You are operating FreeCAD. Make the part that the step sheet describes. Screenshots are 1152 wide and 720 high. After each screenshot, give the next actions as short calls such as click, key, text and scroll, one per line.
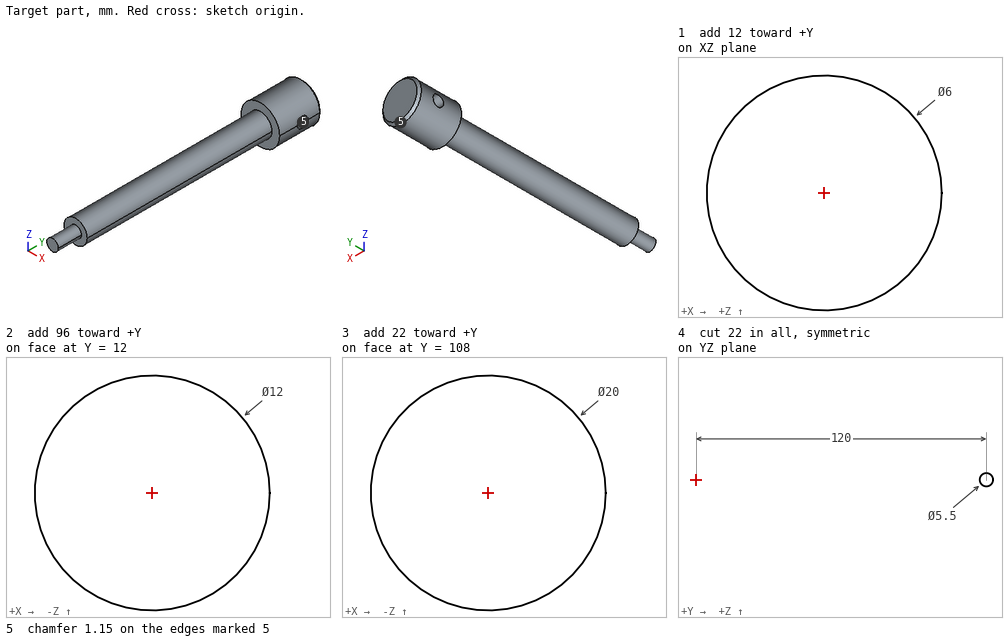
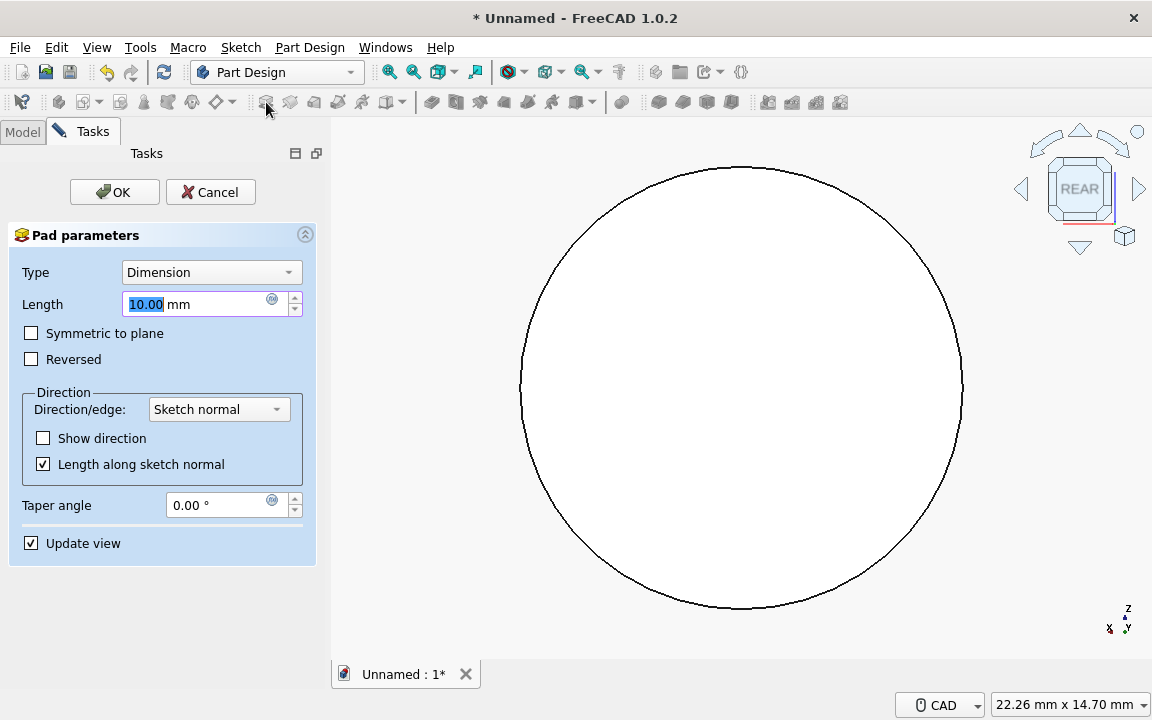
text(96)
key(Tab)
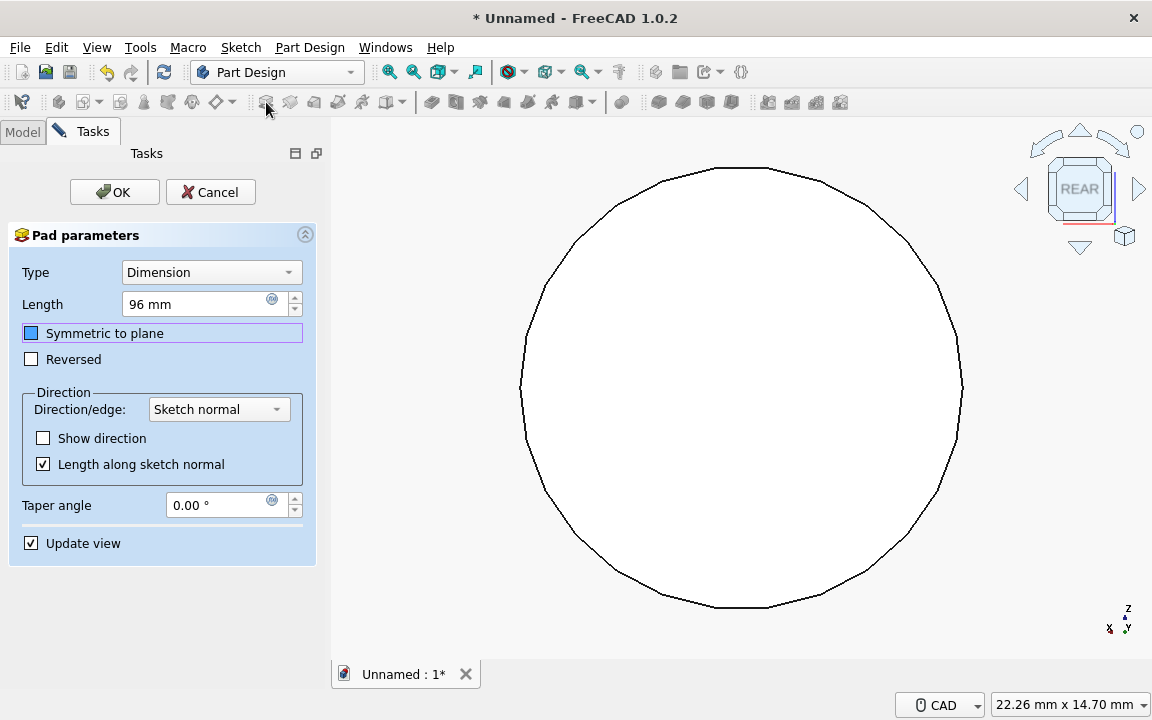
click(115, 192)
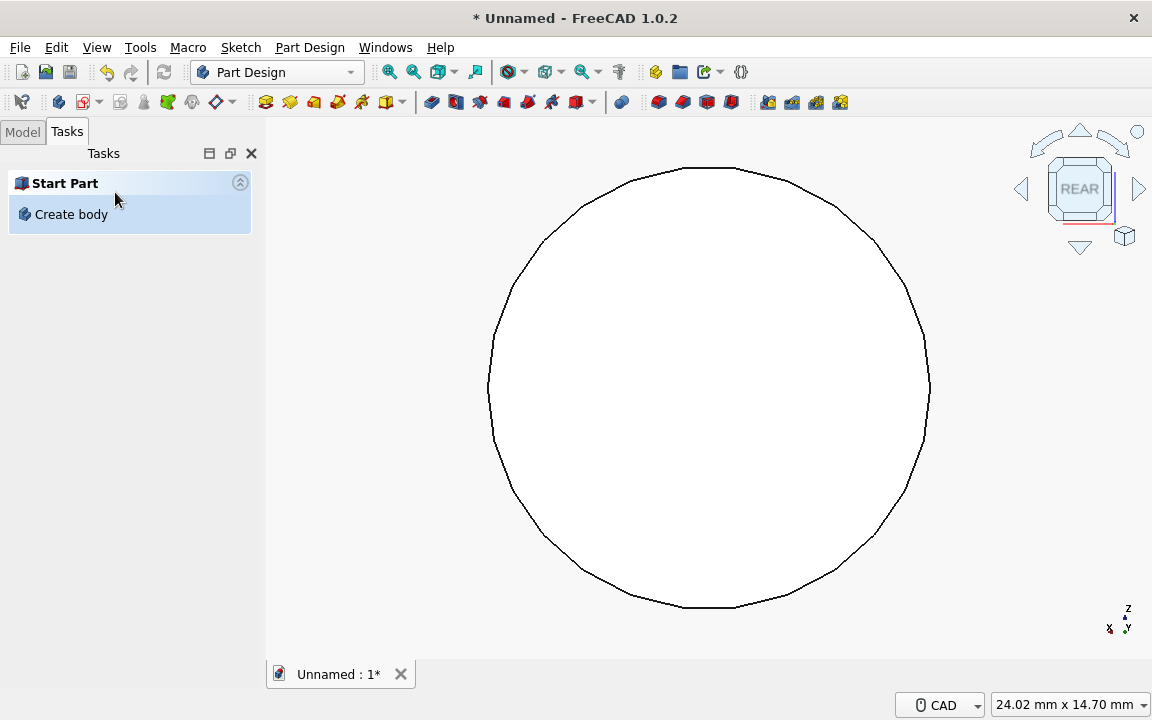
click(709, 387)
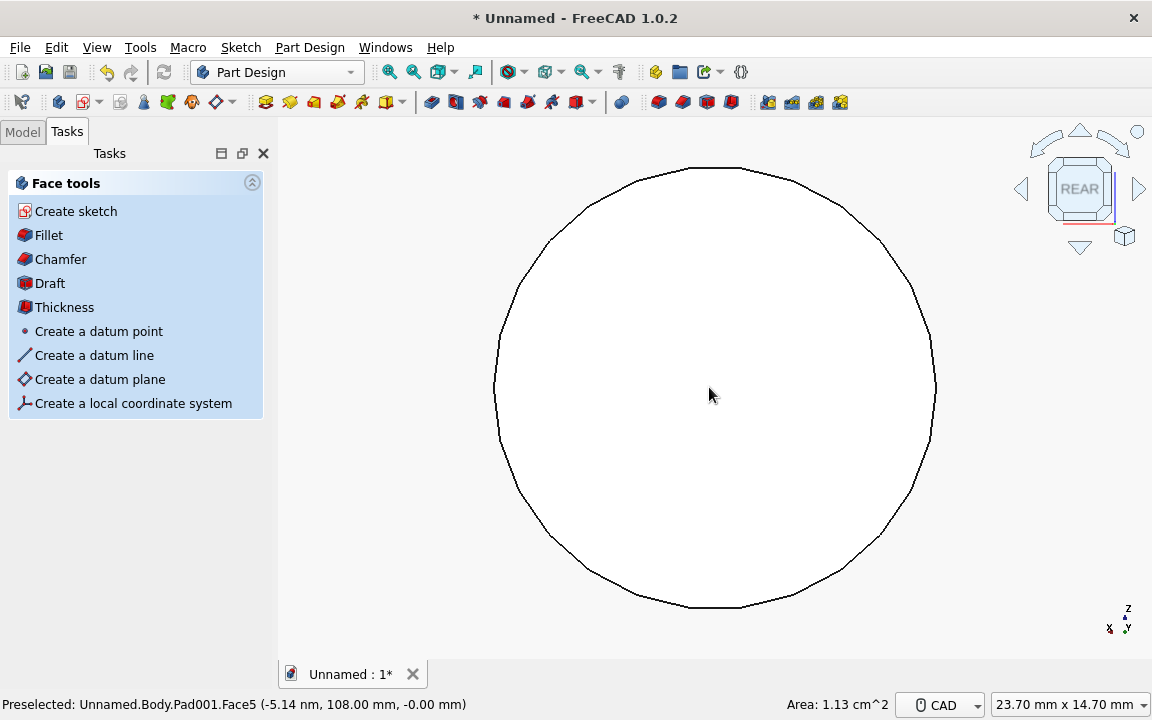
click(84, 102)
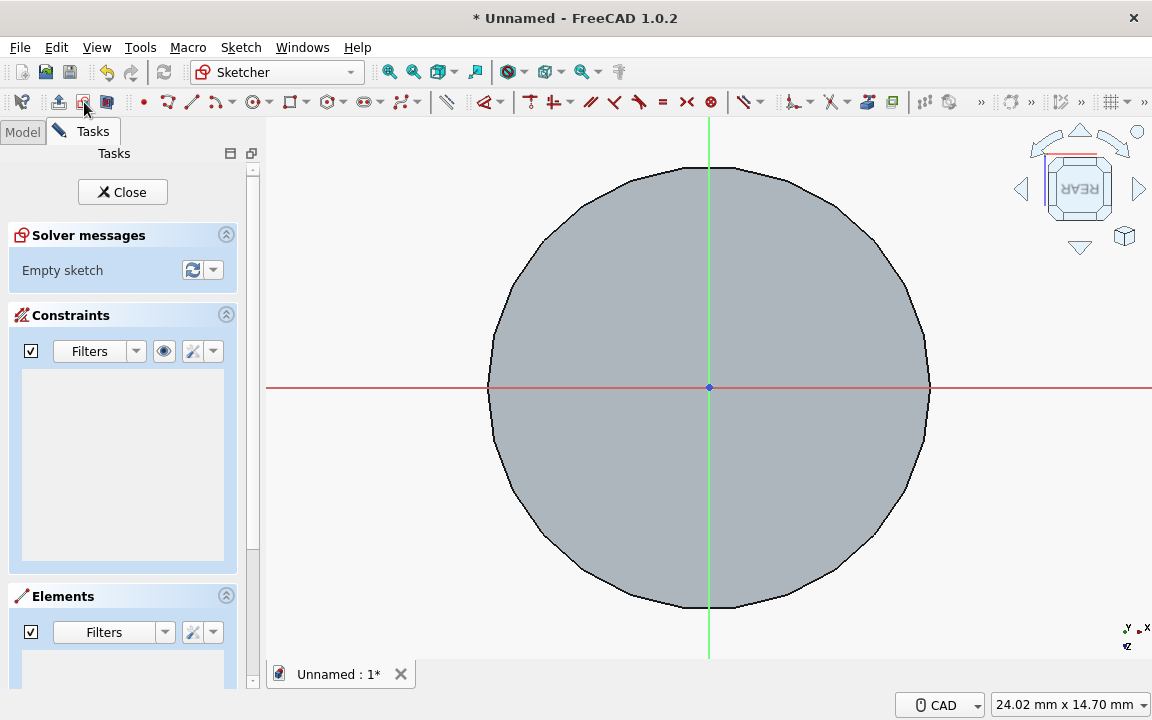
scroll(585, 388, down, 4)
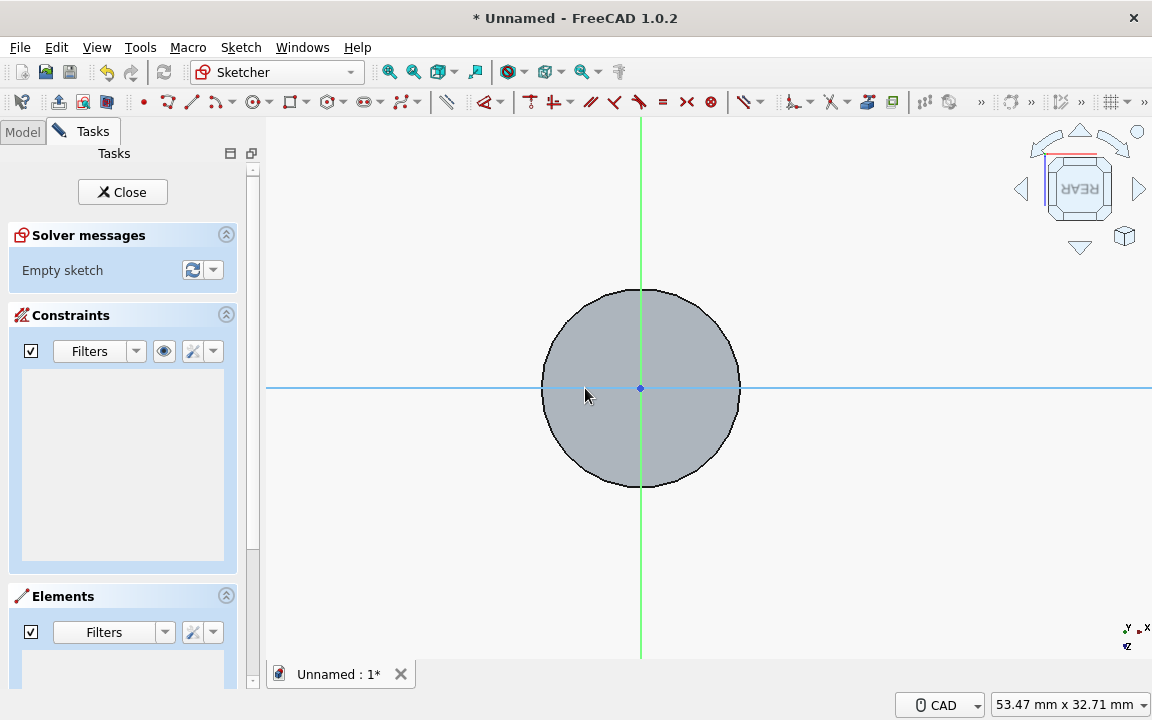
click(254, 102)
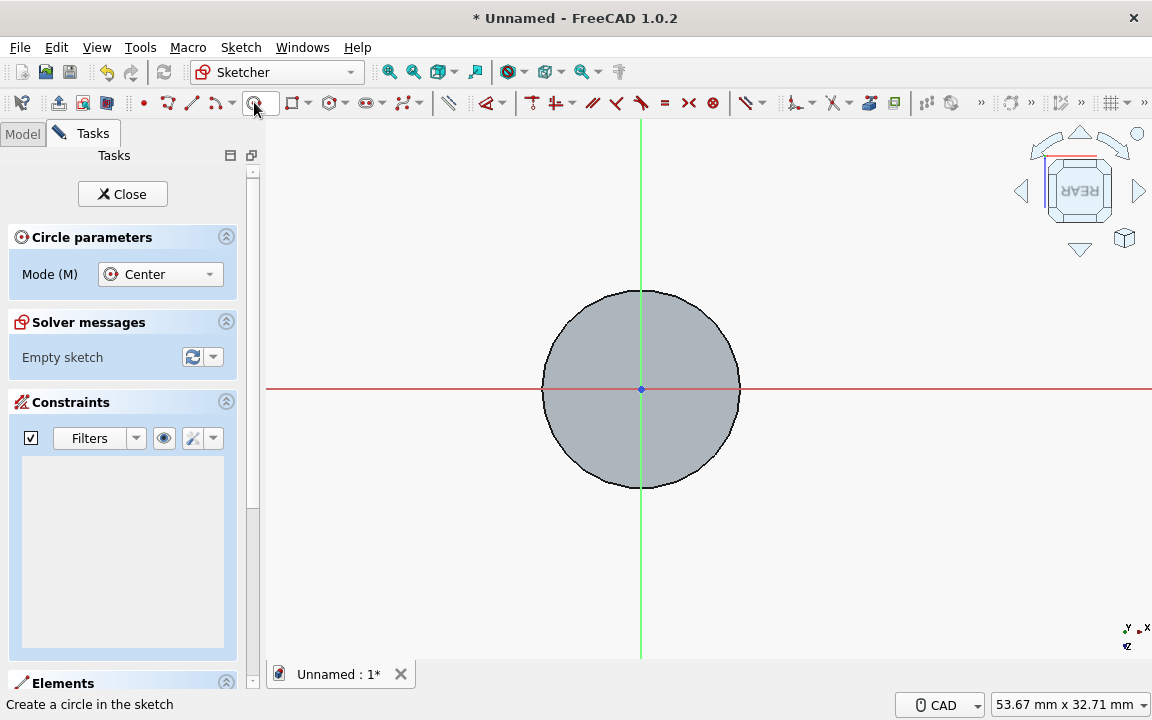
click(641, 389)
move(758, 273)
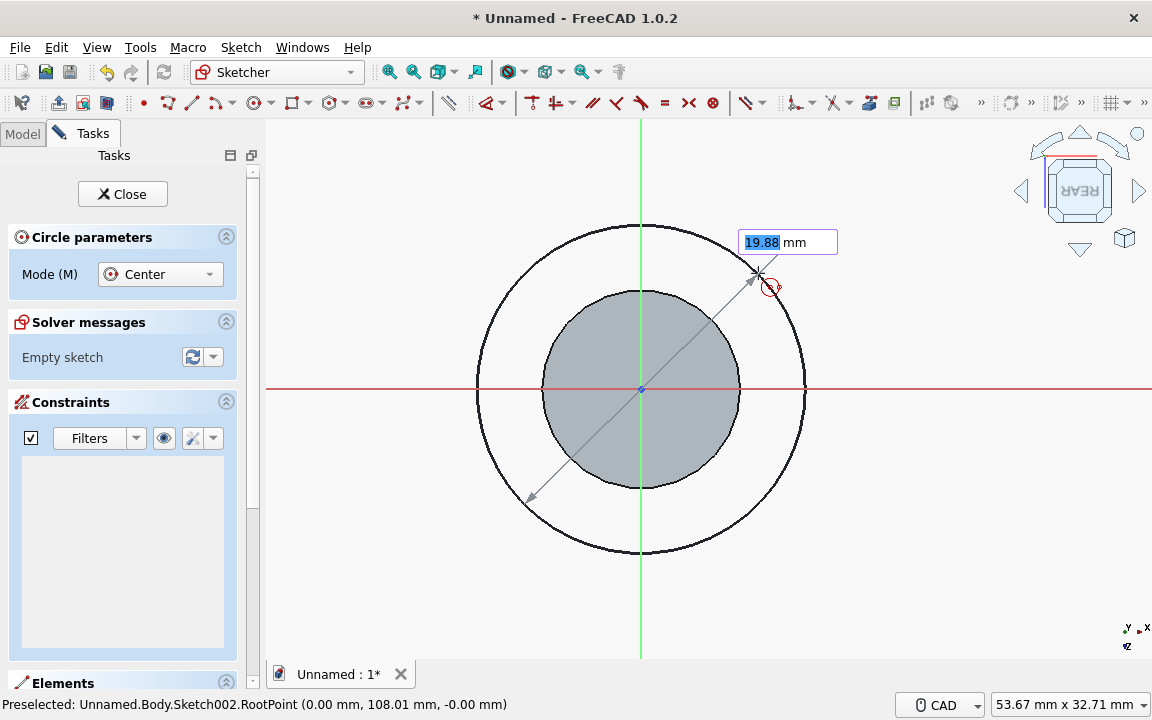
text(20)
key(Return)
key(Escape)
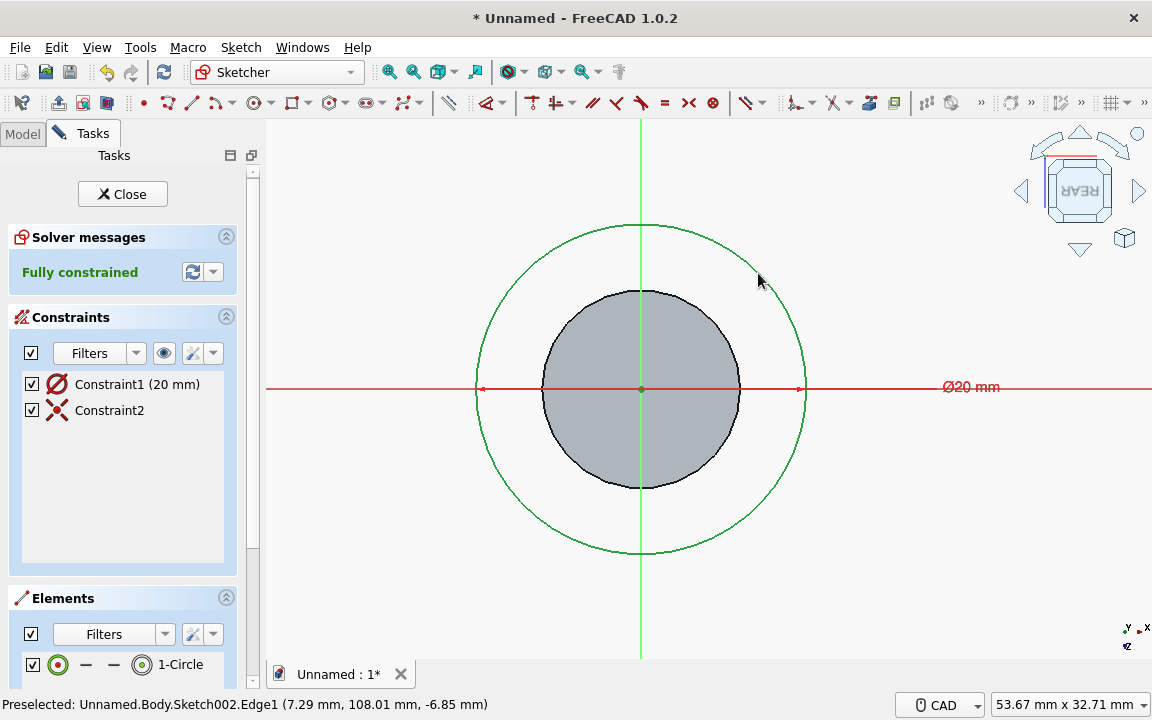
click(123, 194)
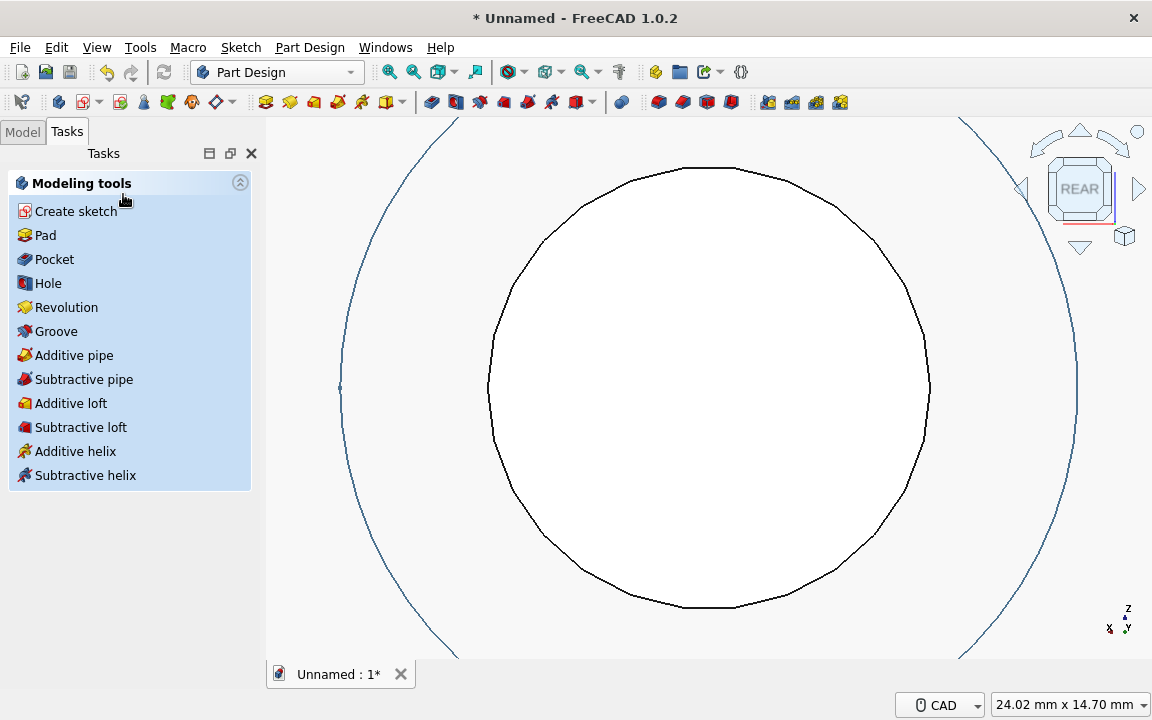
click(266, 102)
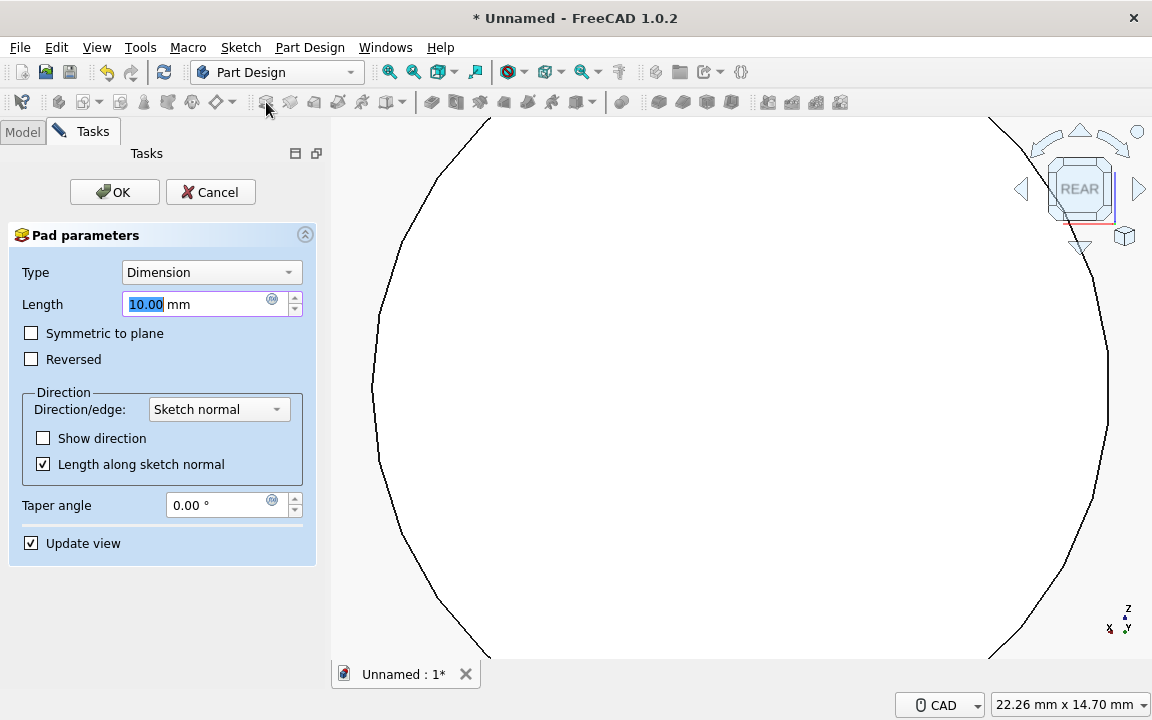
text(22)
key(Tab)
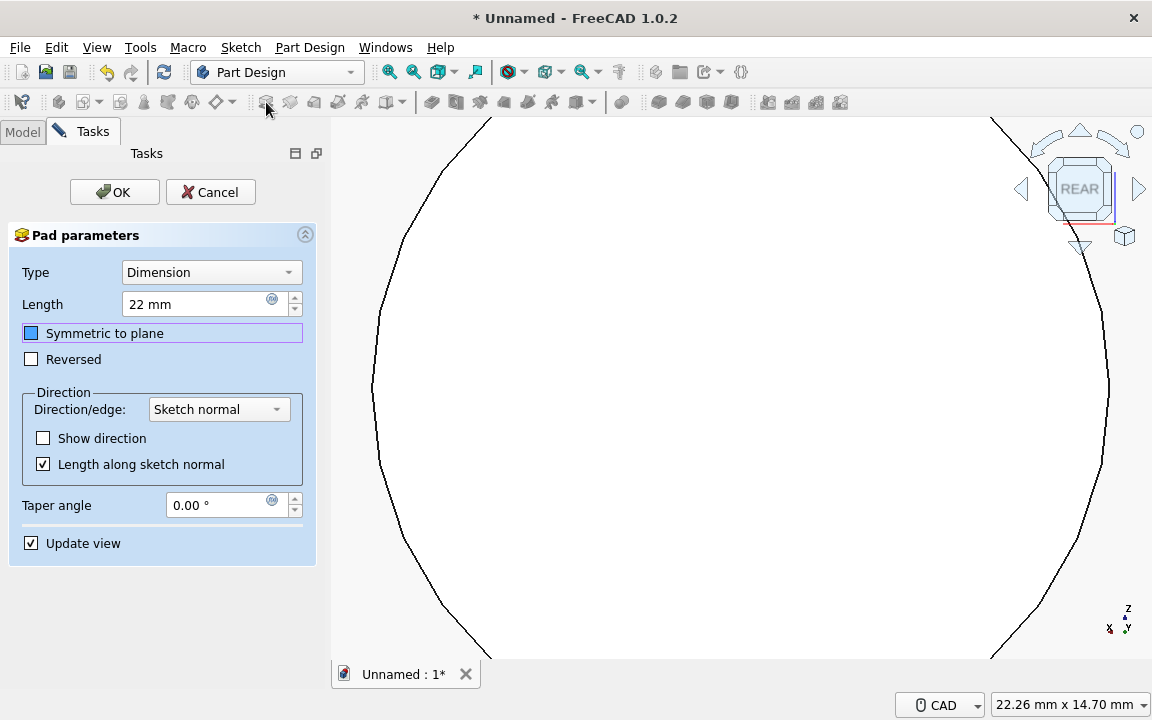
click(115, 192)